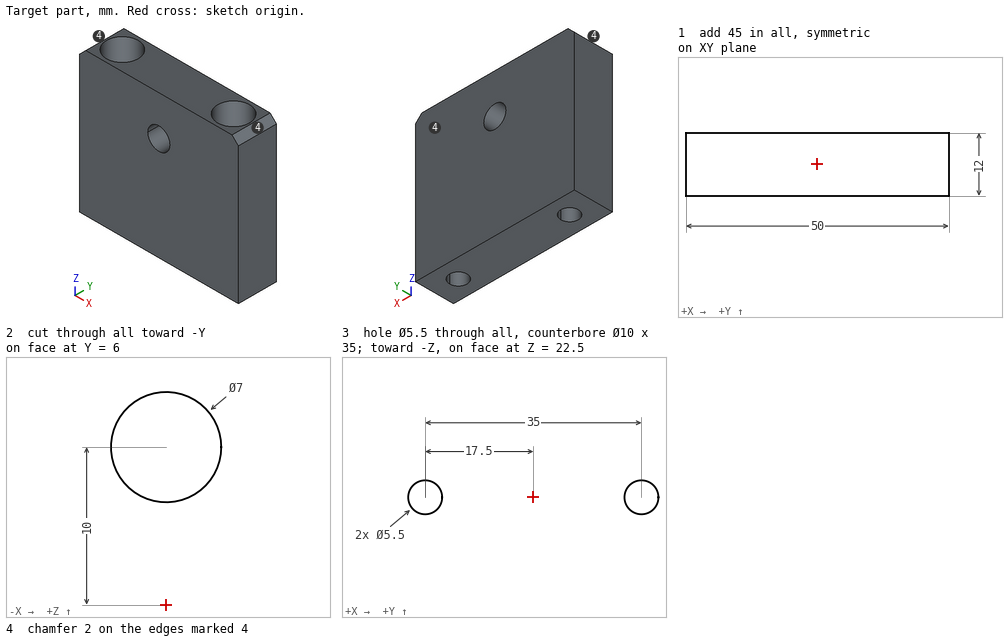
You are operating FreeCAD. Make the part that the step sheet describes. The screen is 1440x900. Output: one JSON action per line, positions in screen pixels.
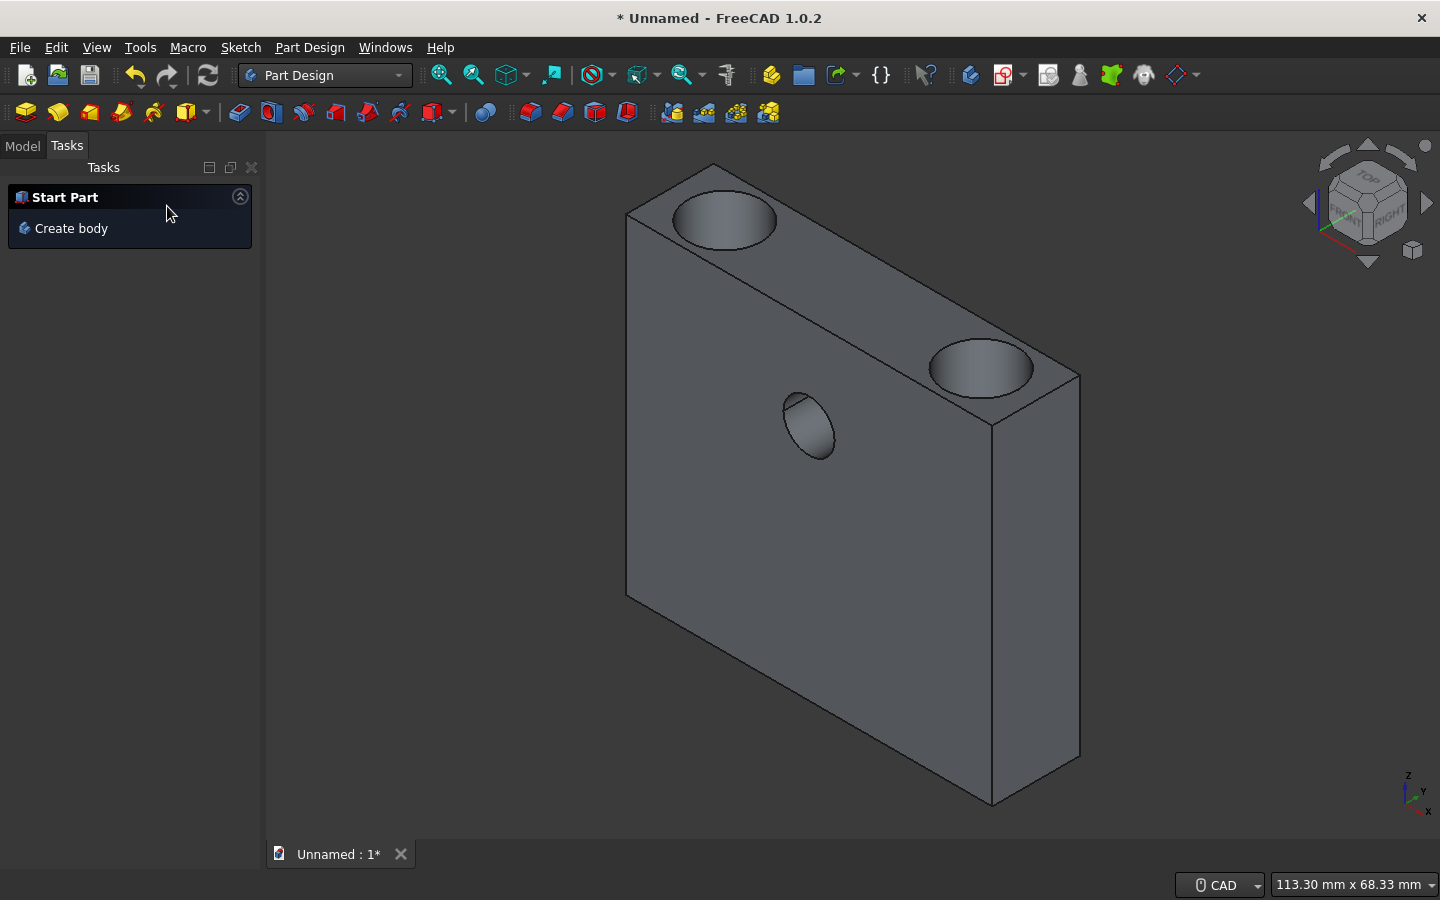
{"action": "left_click", "coordinate": [1036, 399]}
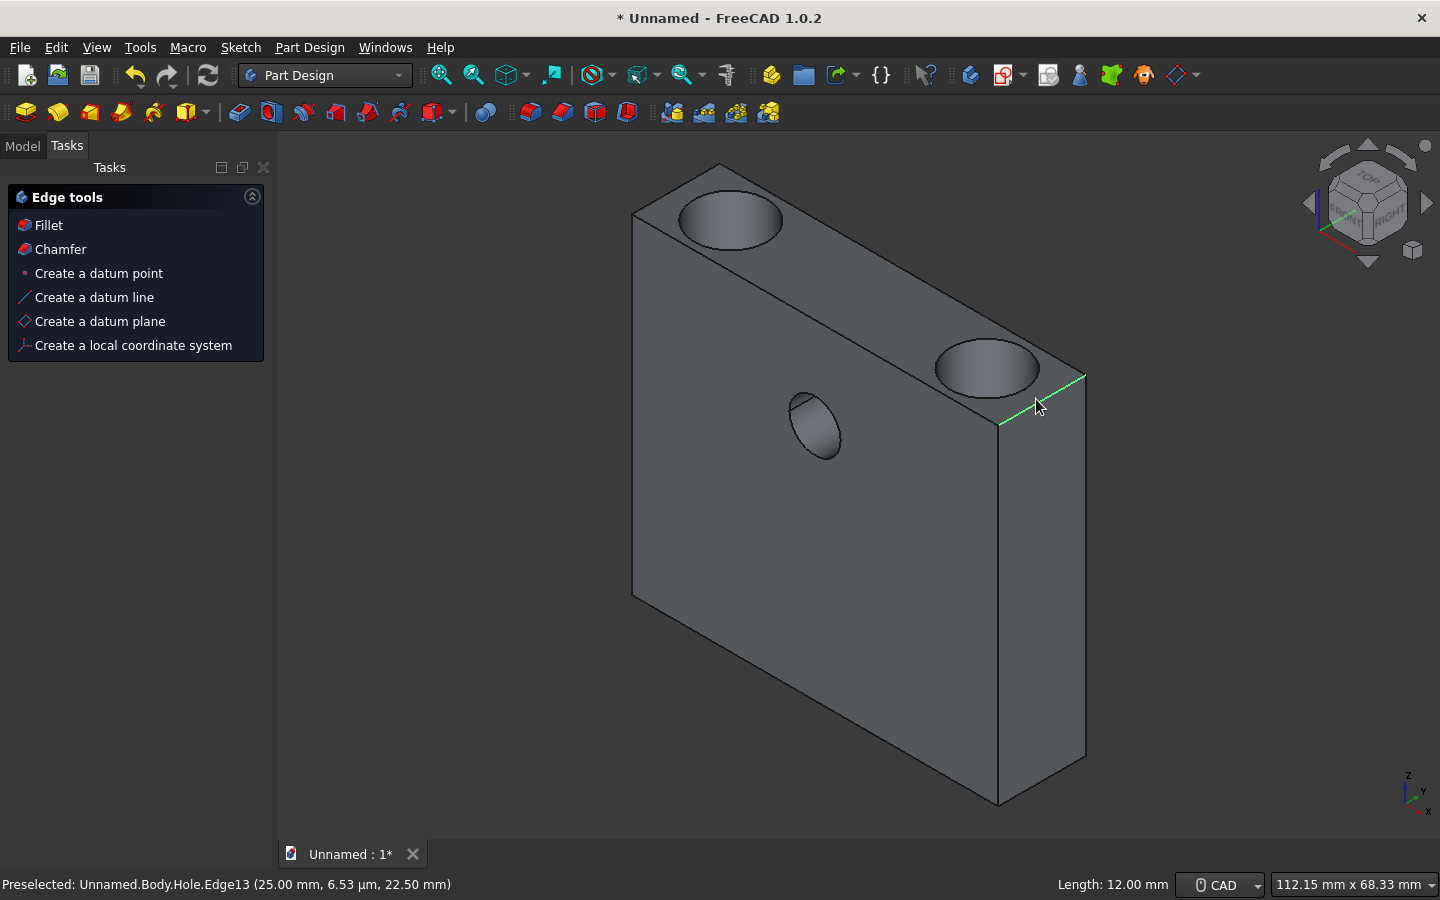
{"action": "key", "text": "2"}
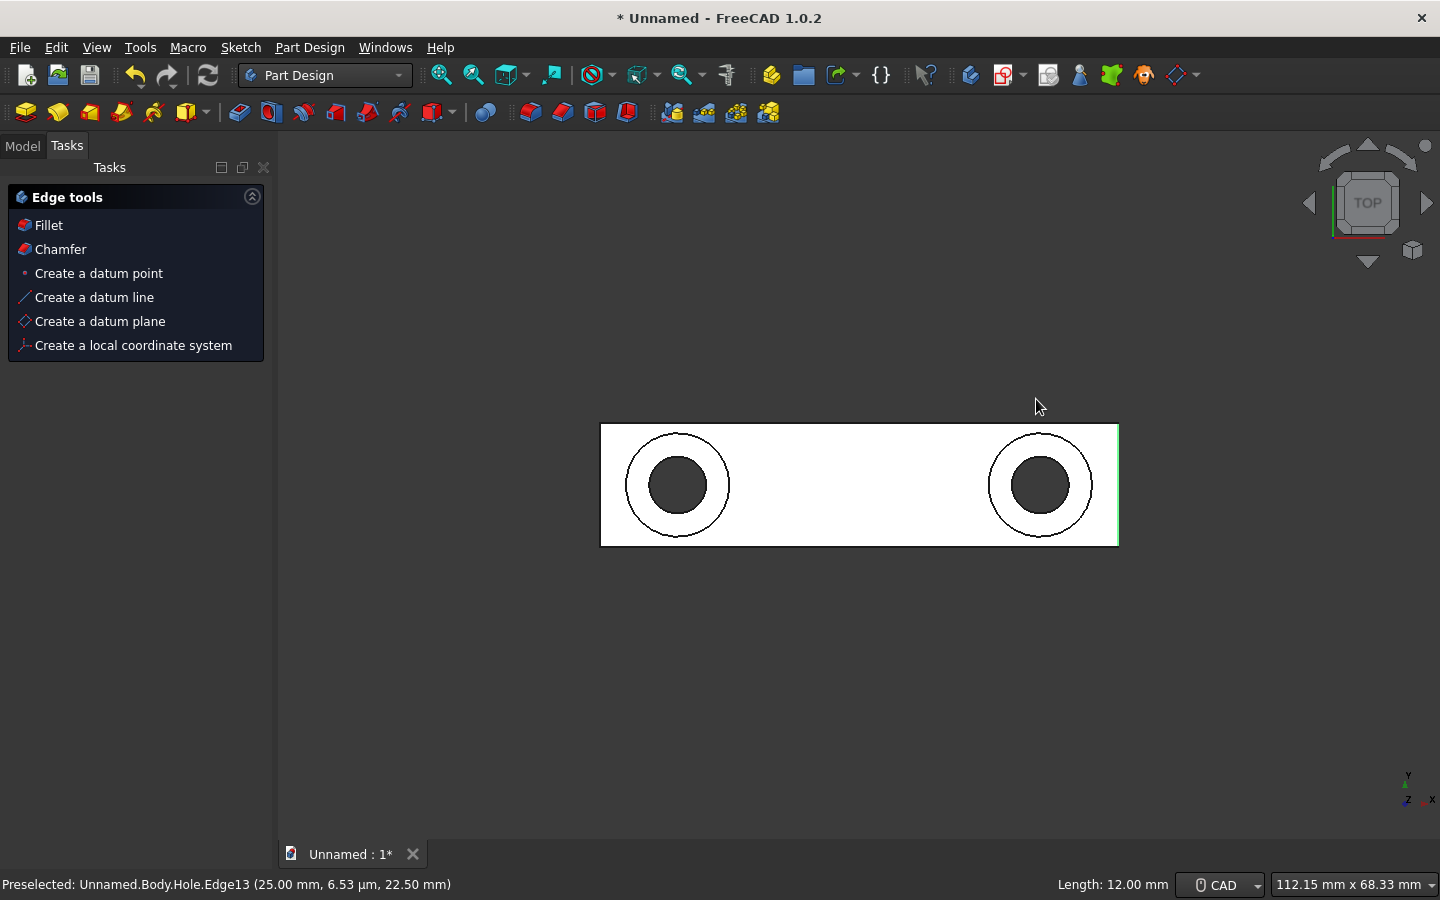
{"action": "left_click", "coordinate": [442, 76]}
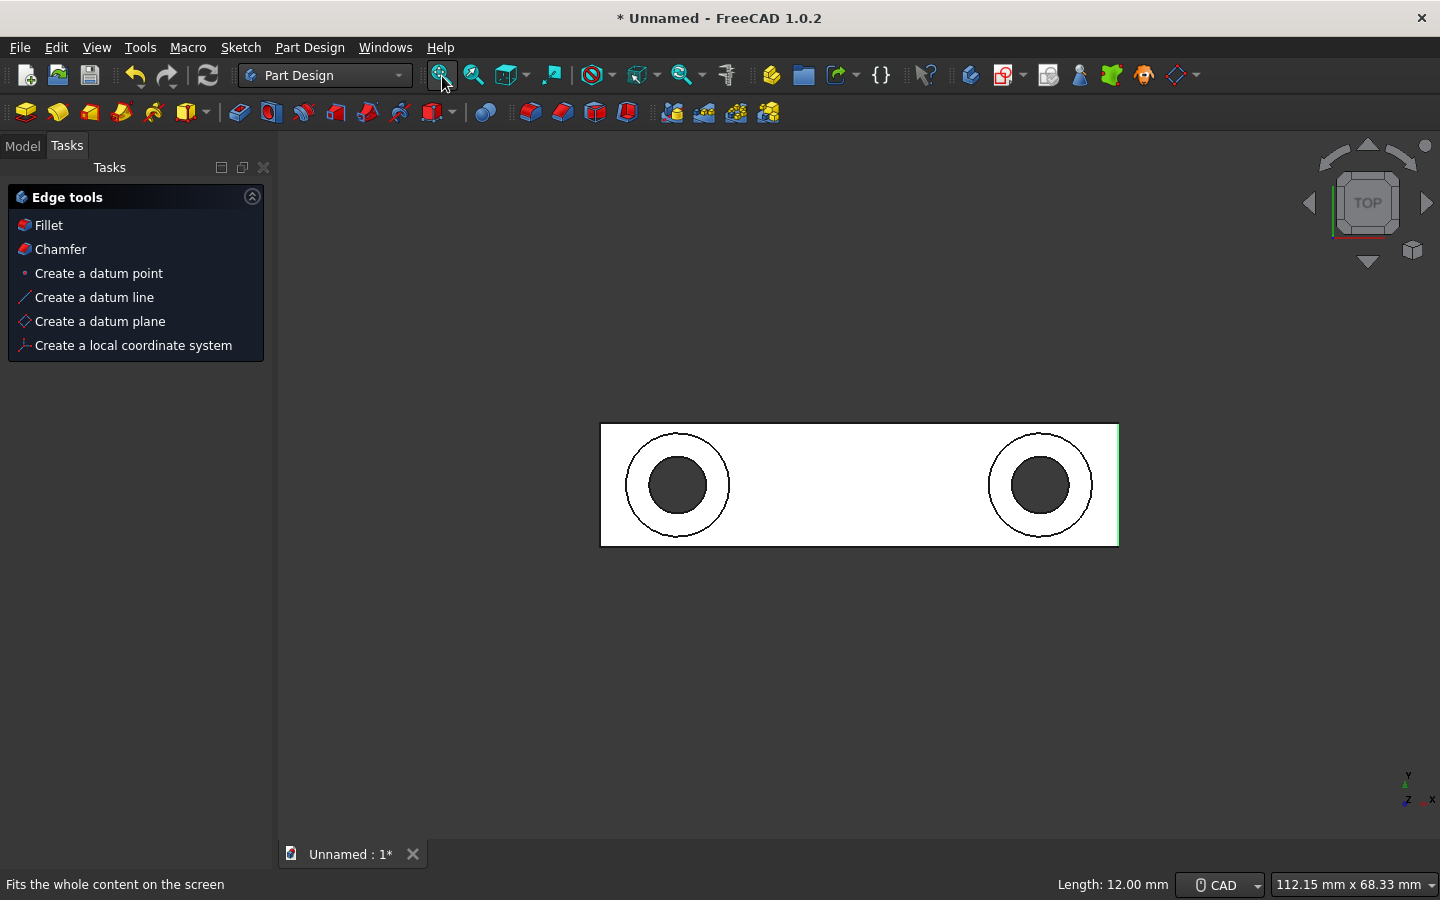
{"action": "left_click", "coordinate": [600, 484], "text": "ctrl"}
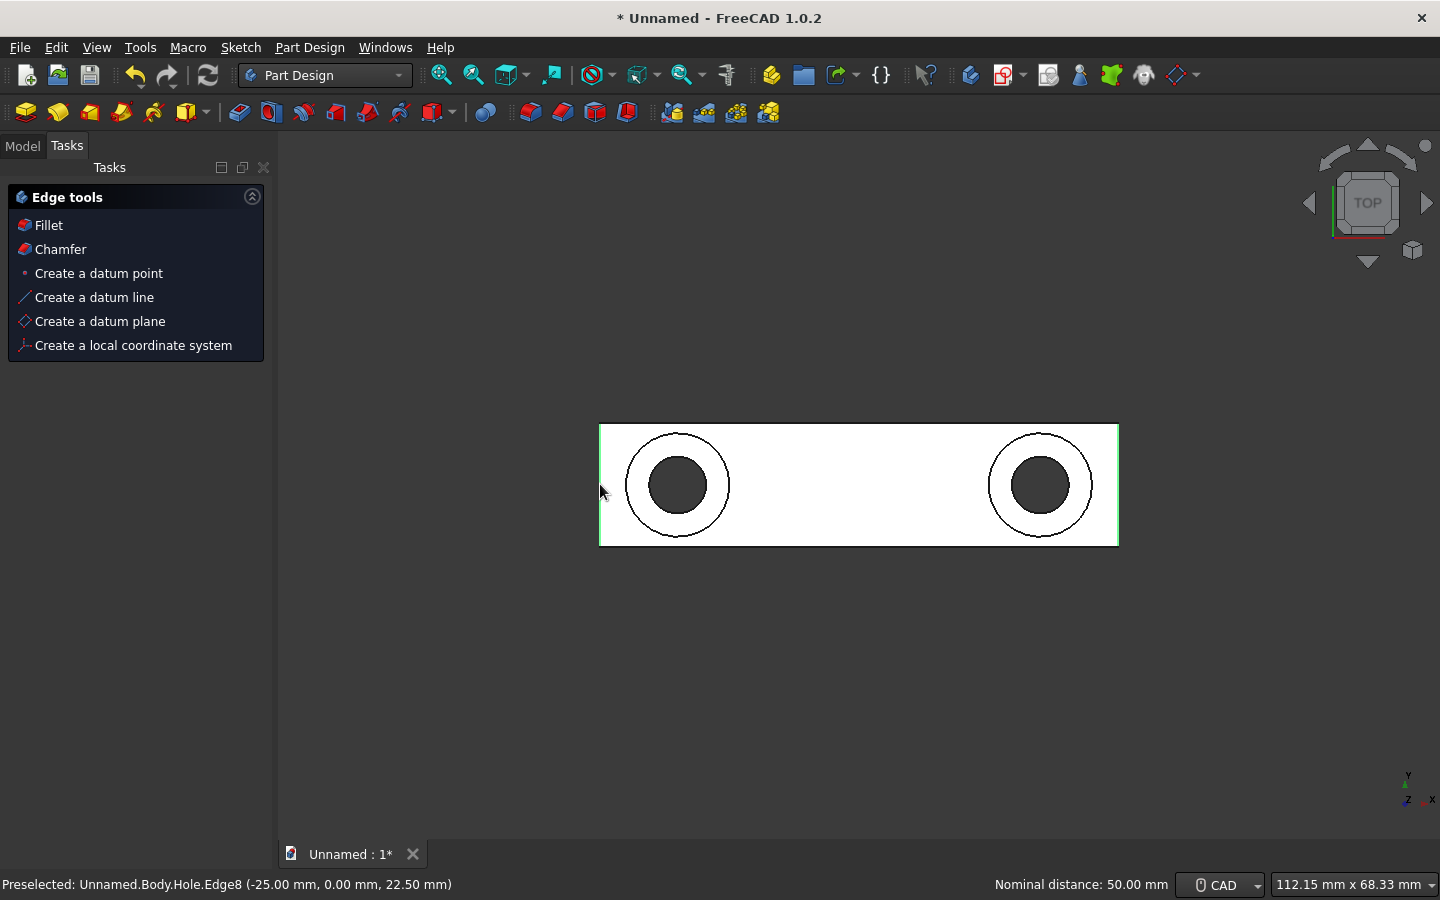
{"action": "left_click", "coordinate": [564, 112]}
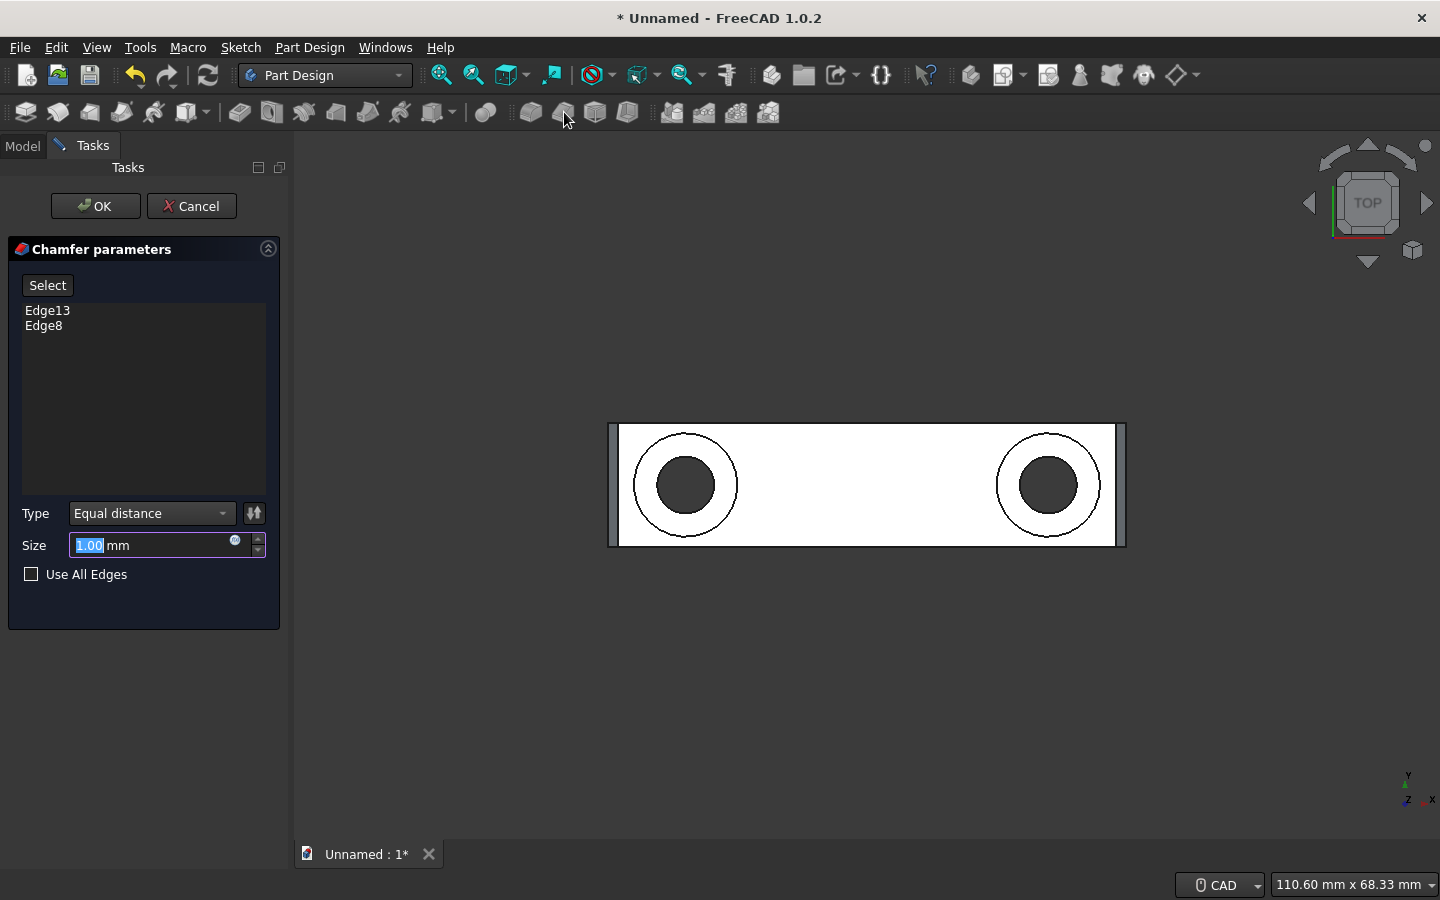
{"action": "type", "text": "2"}
{"action": "key", "text": "Tab"}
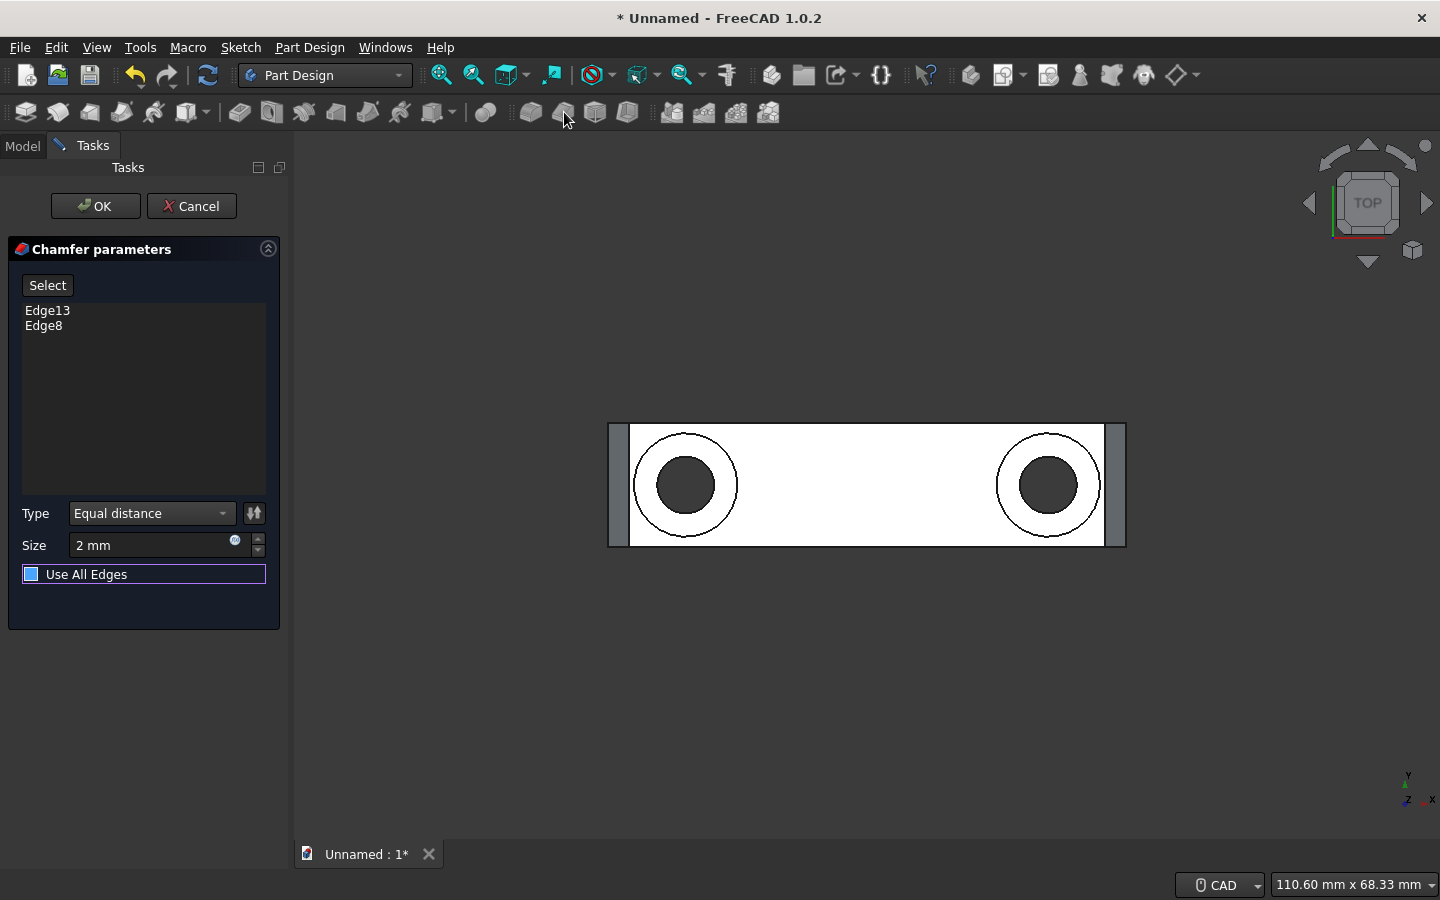
{"action": "left_click", "coordinate": [96, 206]}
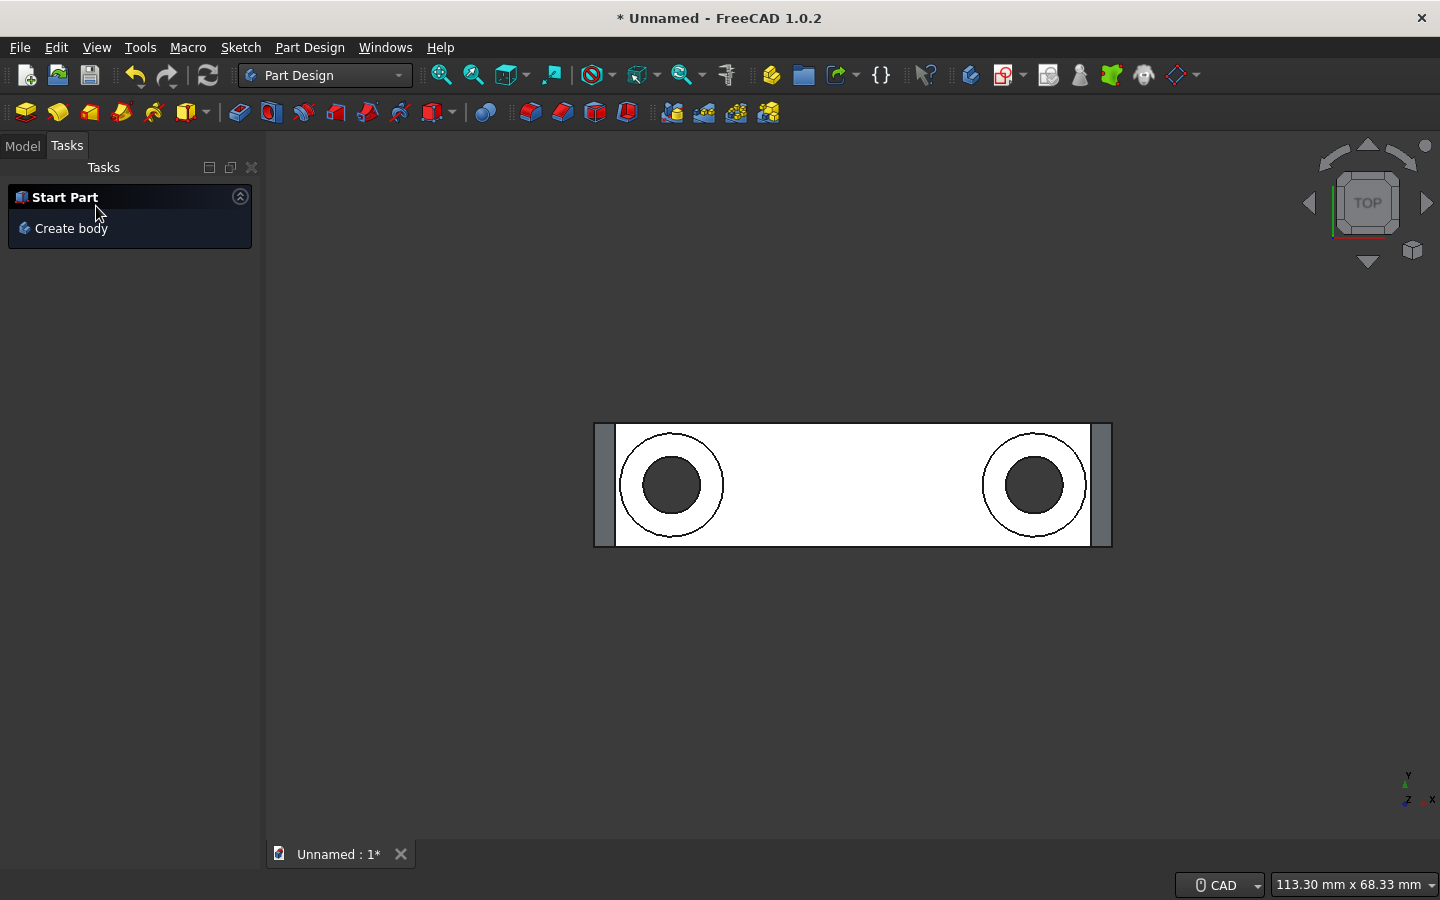
{"action": "key", "text": "0"}